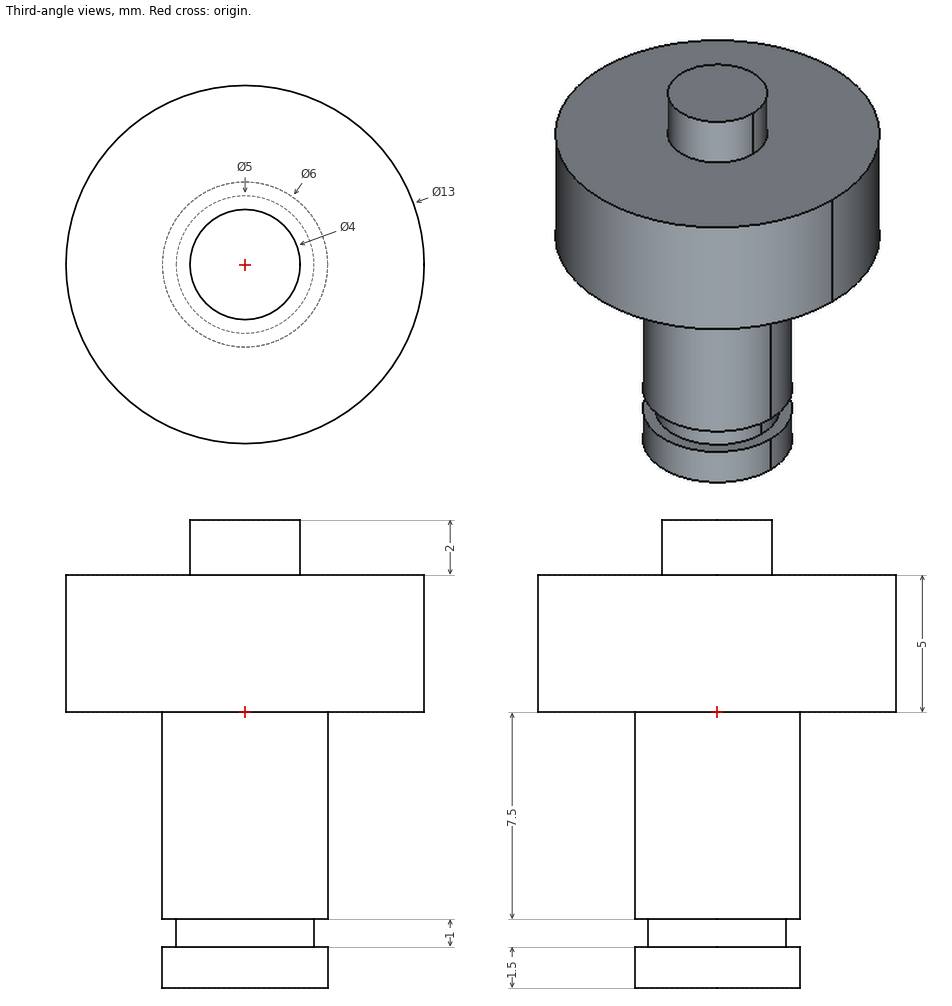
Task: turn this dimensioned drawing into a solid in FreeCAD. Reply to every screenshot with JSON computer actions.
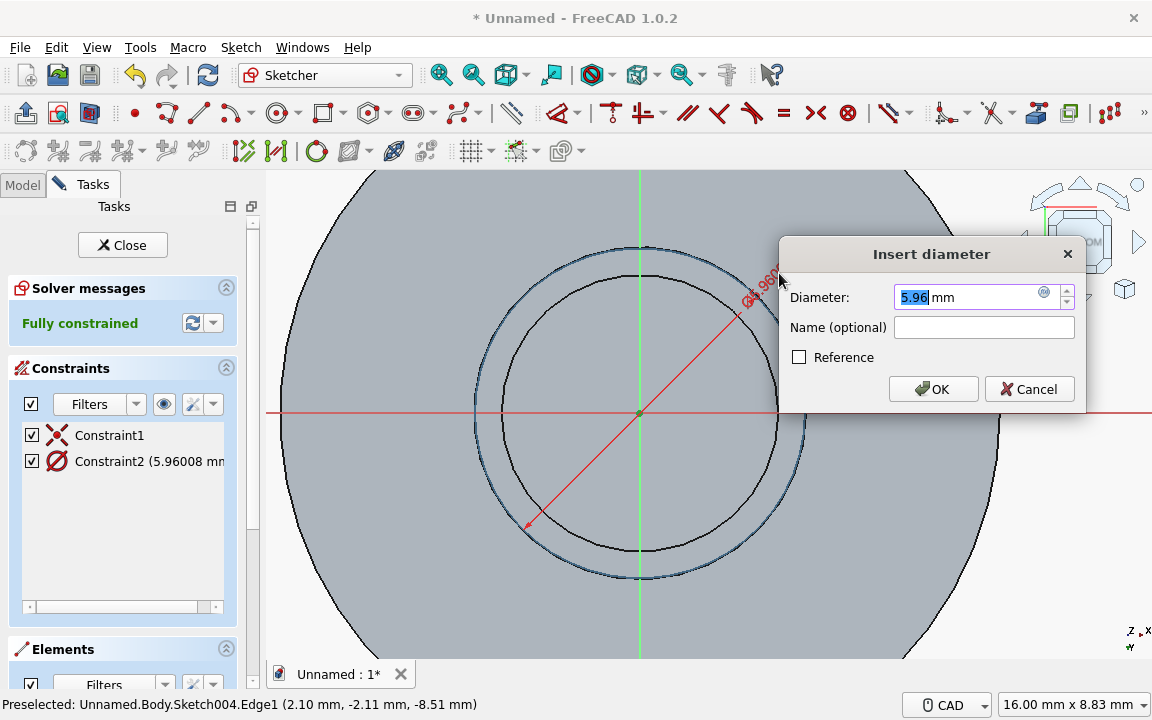
{"action": "type", "text": "6"}
{"action": "key", "text": "Return"}
{"action": "key", "text": "Escape"}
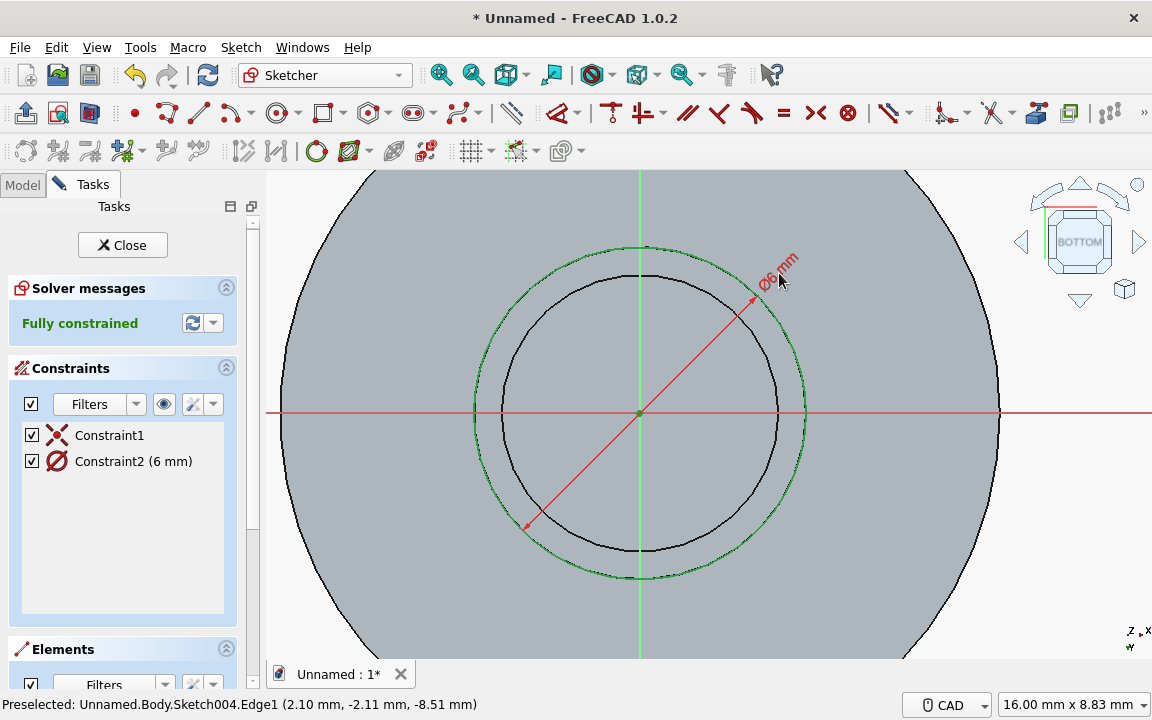
{"action": "left_click", "coordinate": [123, 245]}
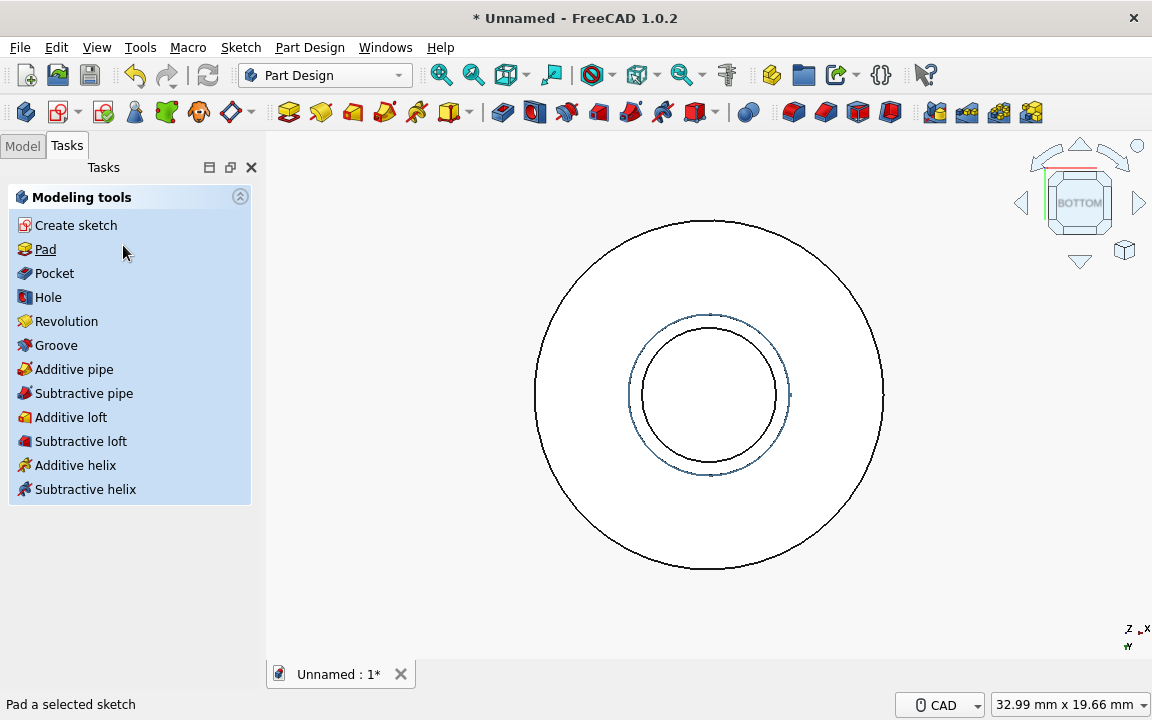
{"action": "left_click", "coordinate": [290, 112]}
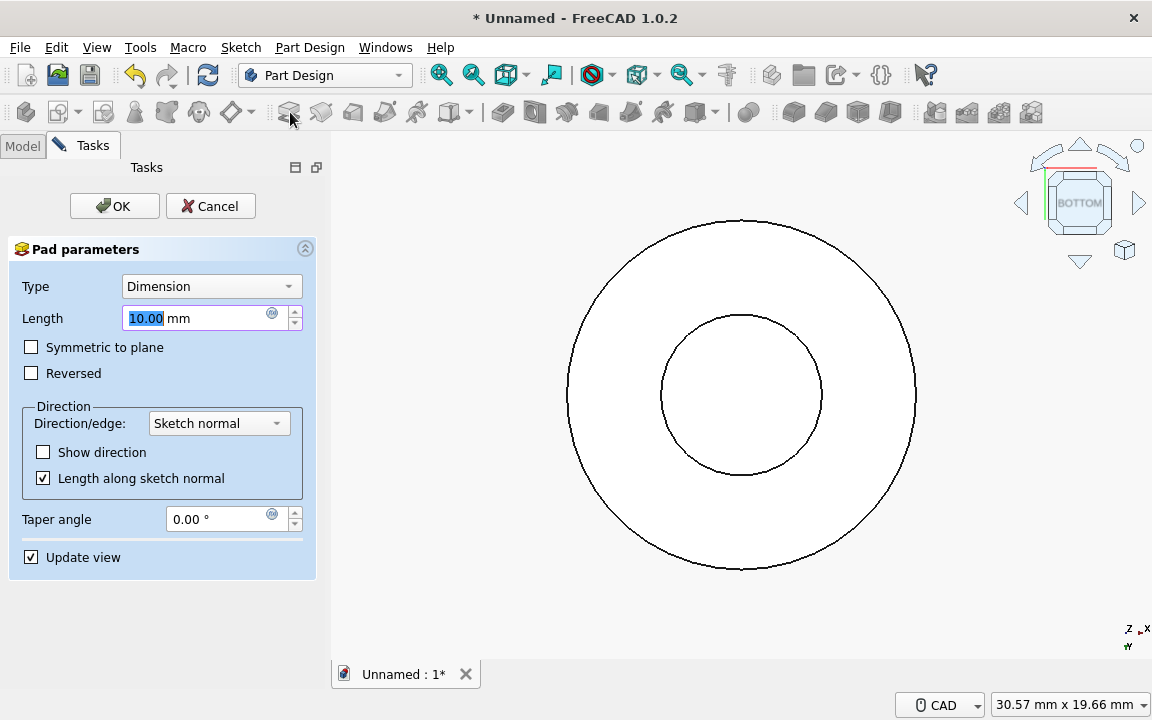
{"action": "type", "text": "1.5"}
{"action": "key", "text": "Tab"}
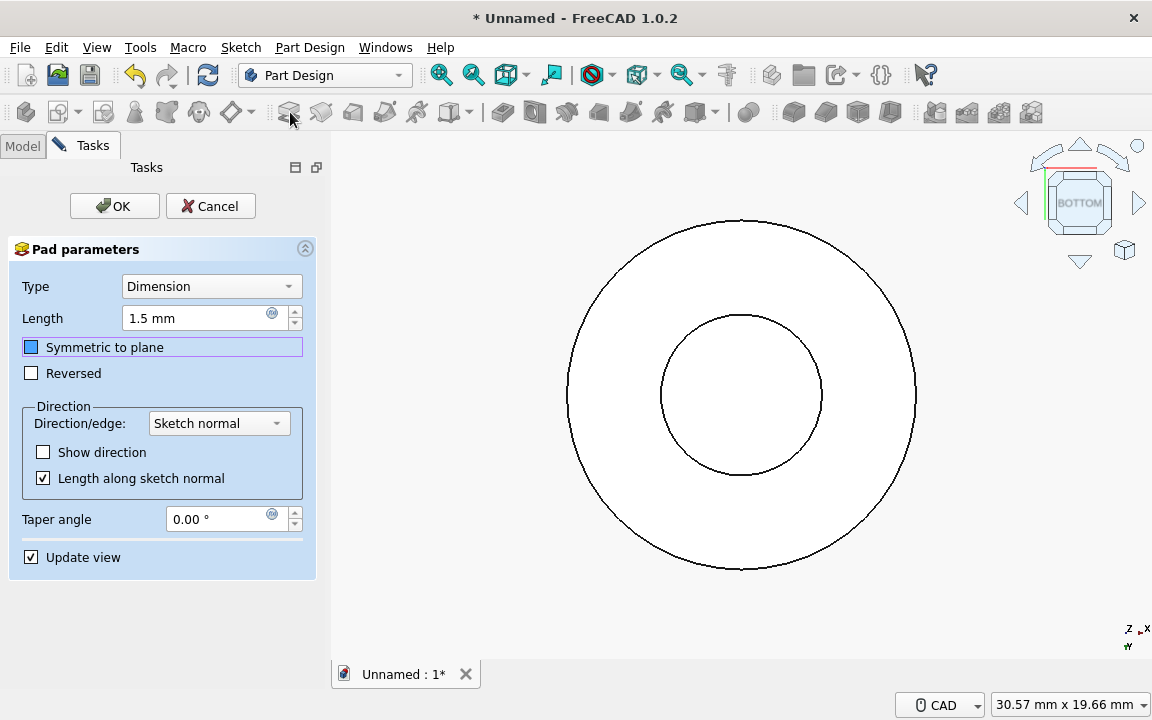
{"action": "left_click", "coordinate": [115, 206]}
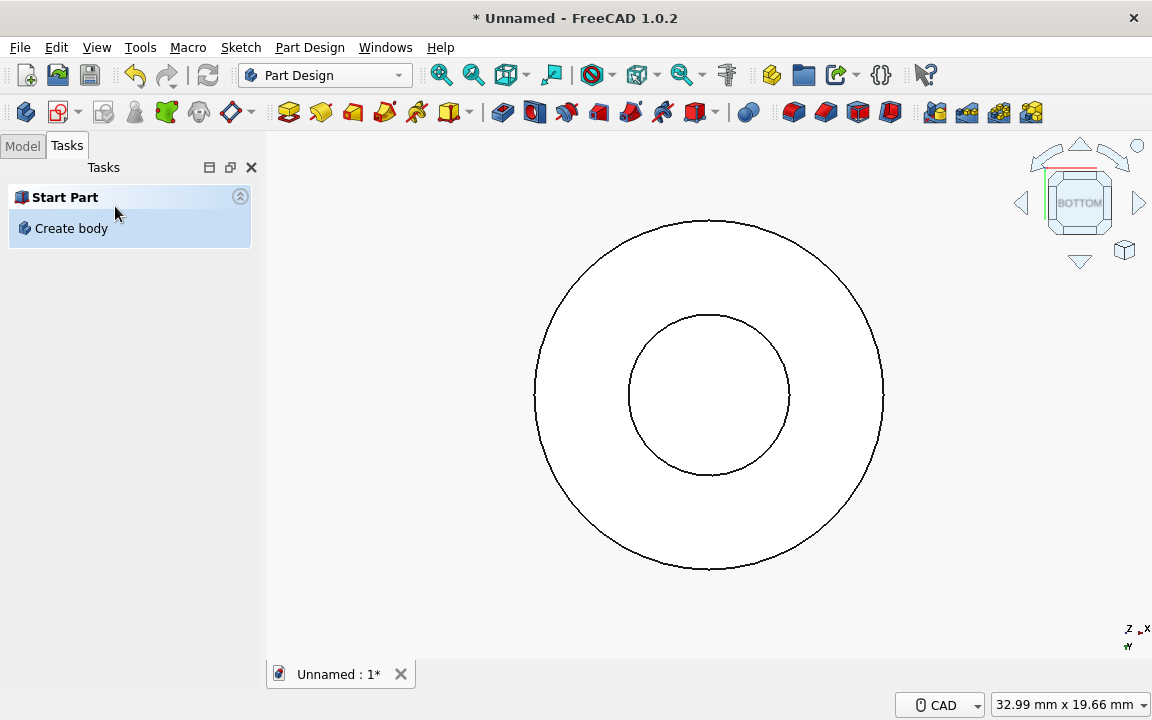
{"action": "key", "text": "0"}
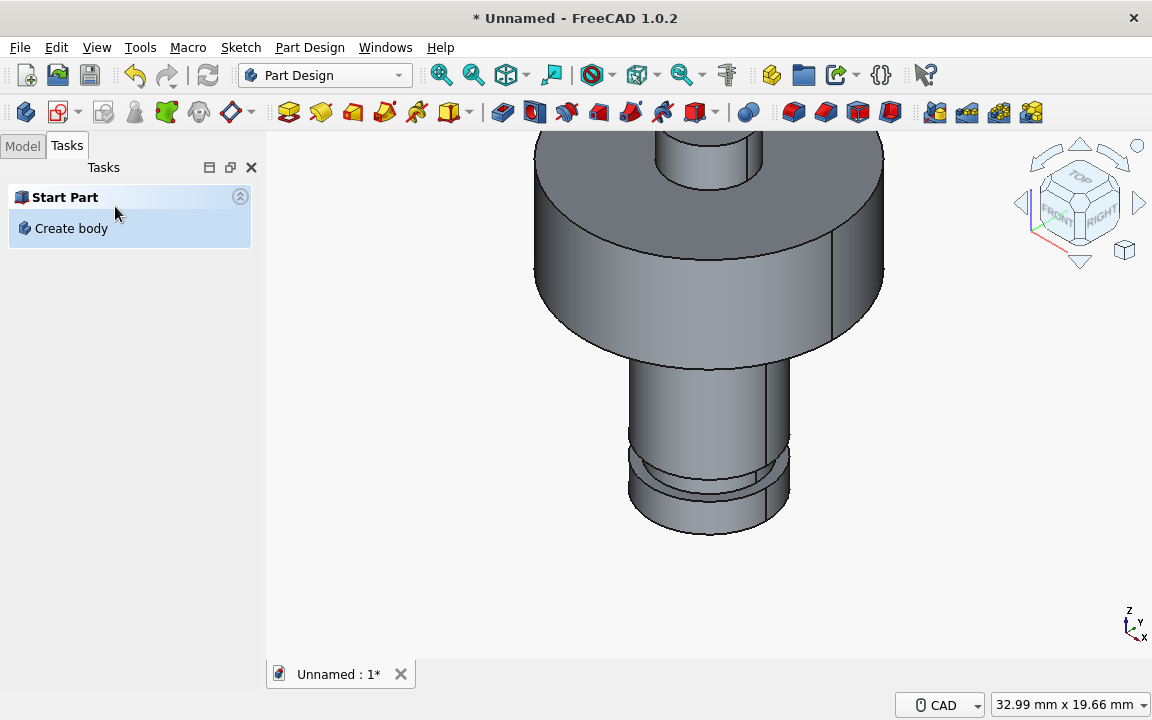
{"action": "key", "text": "v f"}